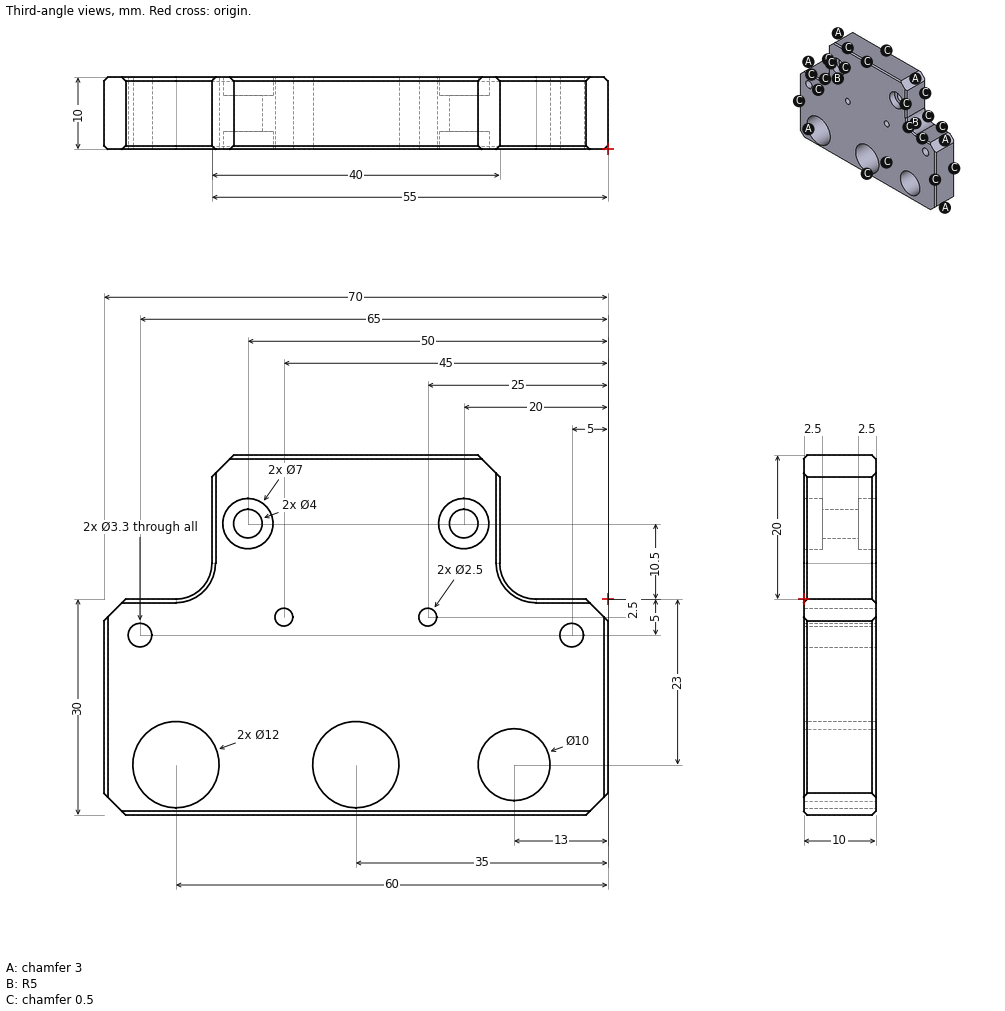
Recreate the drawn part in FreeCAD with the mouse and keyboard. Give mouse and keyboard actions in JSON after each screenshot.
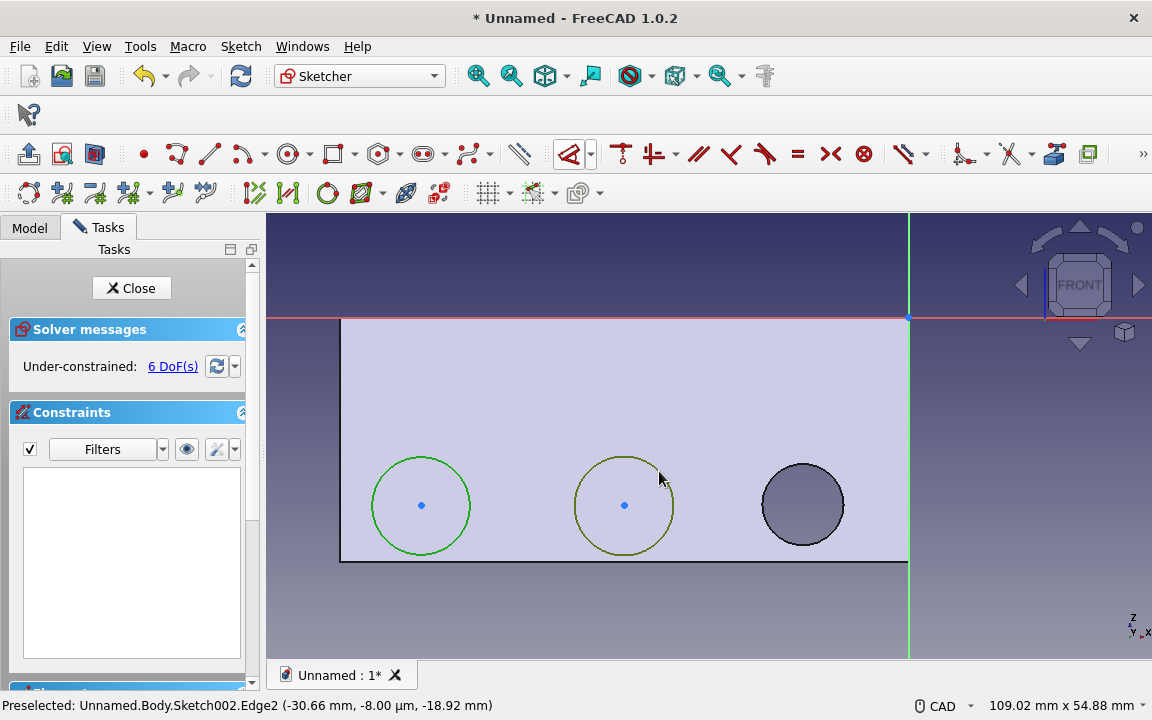
{"action": "left_click", "coordinate": [798, 154]}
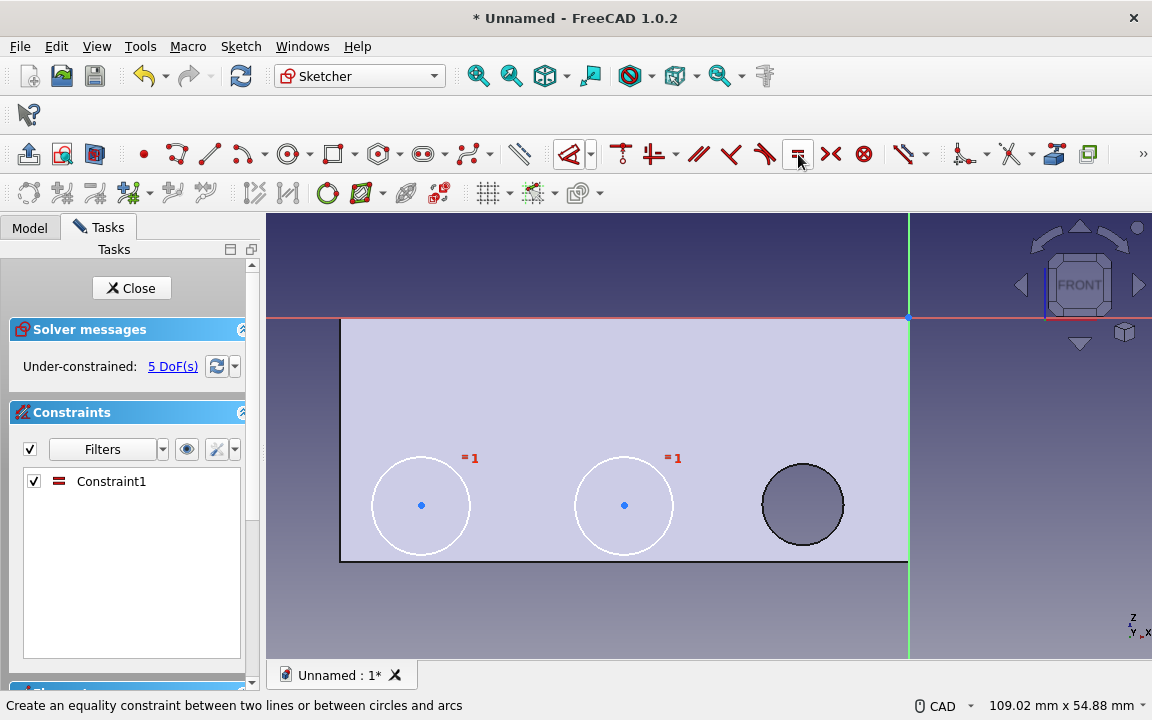
{"action": "left_click", "coordinate": [421, 506]}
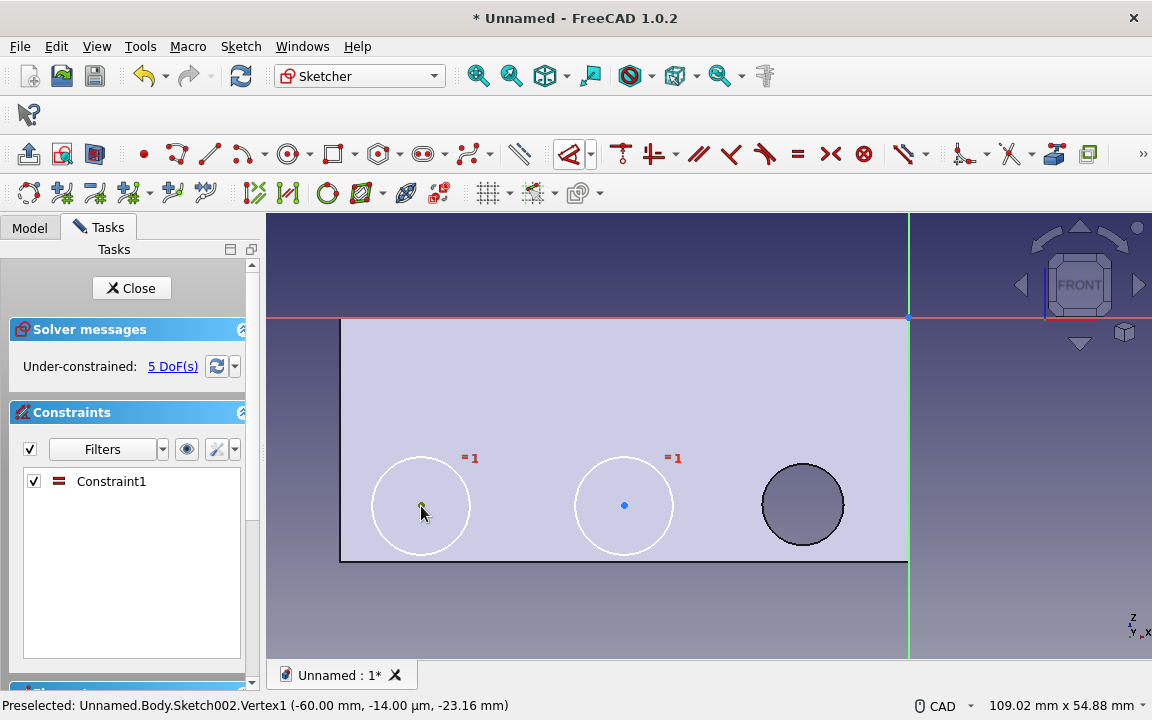
{"action": "left_click", "coordinate": [624, 506]}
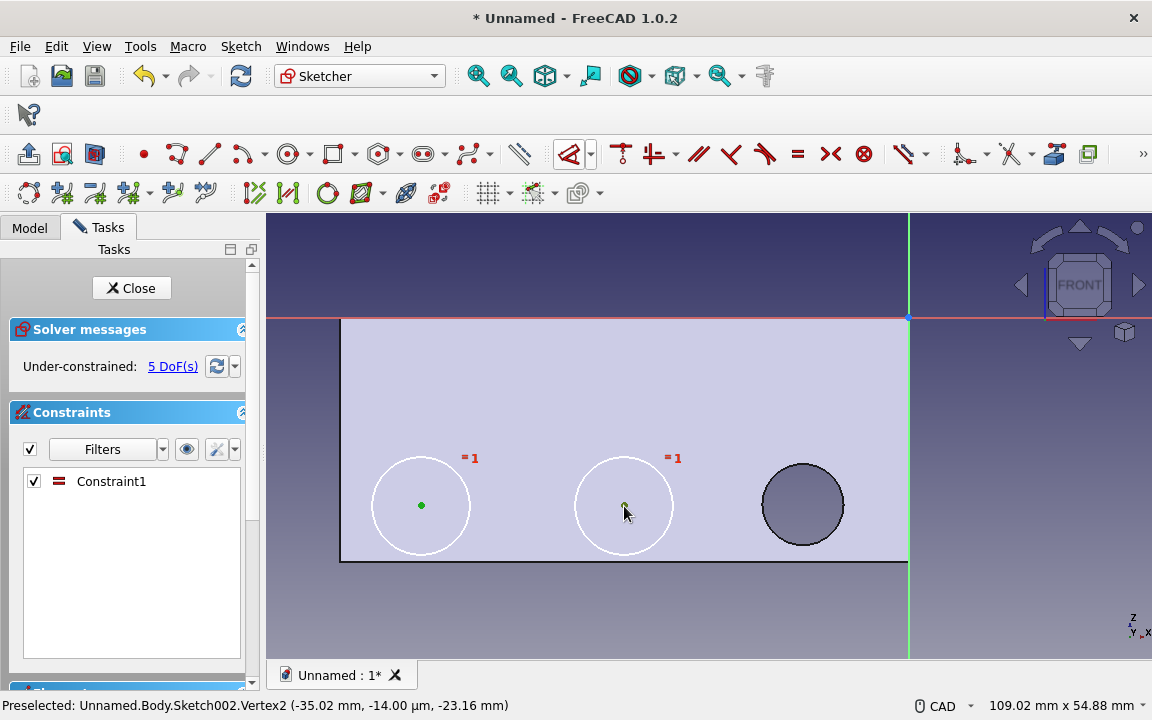
{"action": "left_click", "coordinate": [676, 154]}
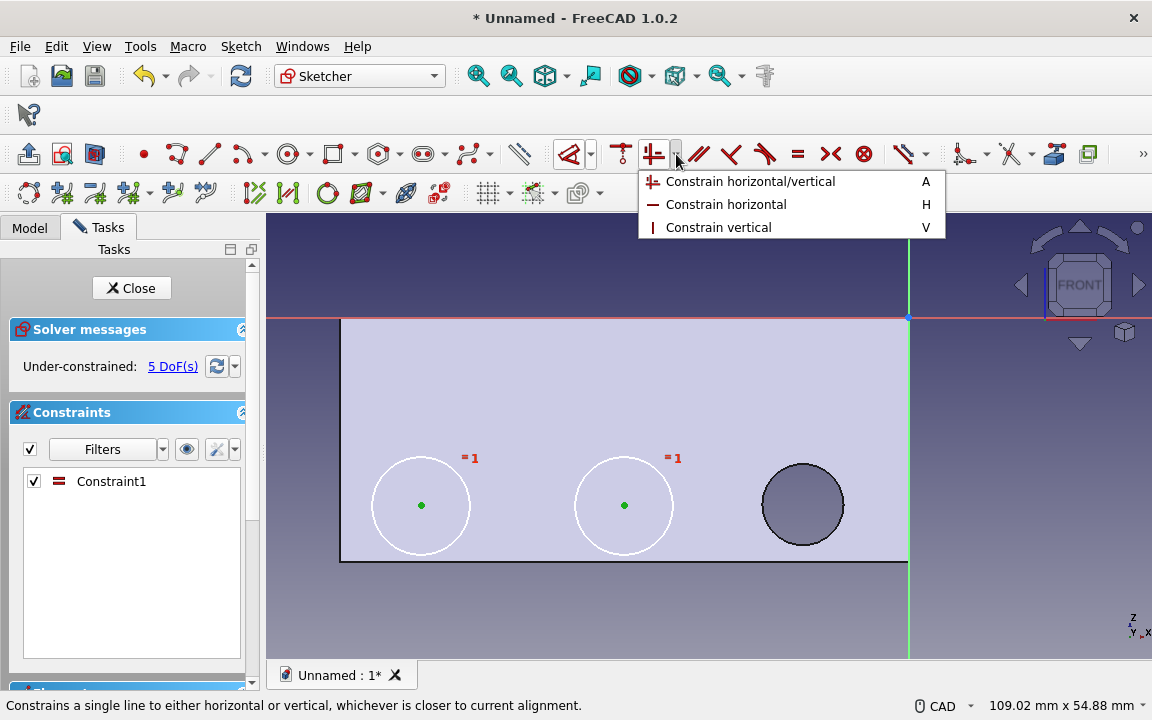
{"action": "left_click", "coordinate": [792, 204]}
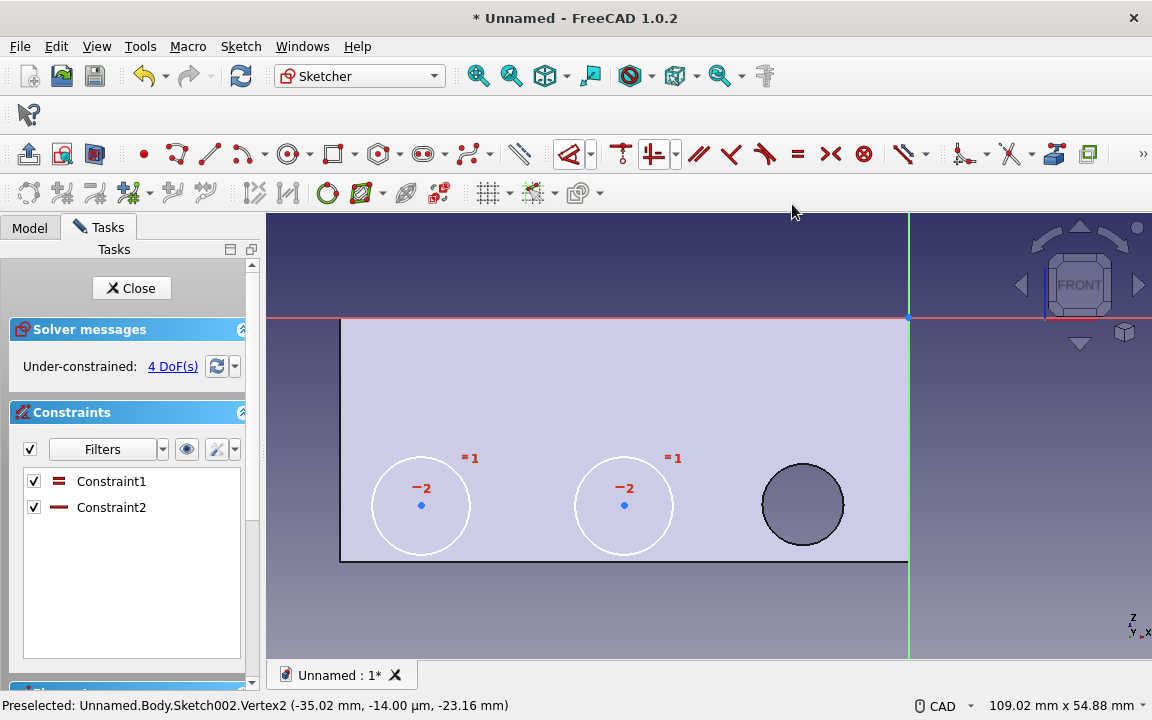
{"action": "left_click", "coordinate": [455, 471]}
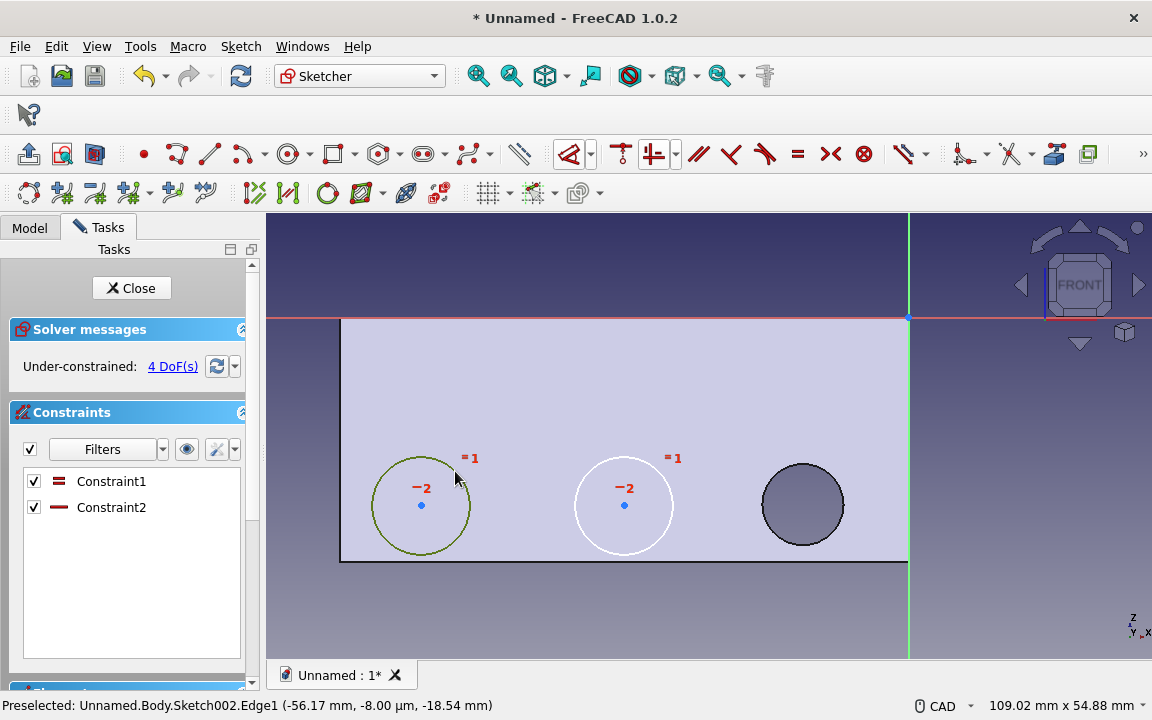
{"action": "left_click", "coordinate": [590, 154]}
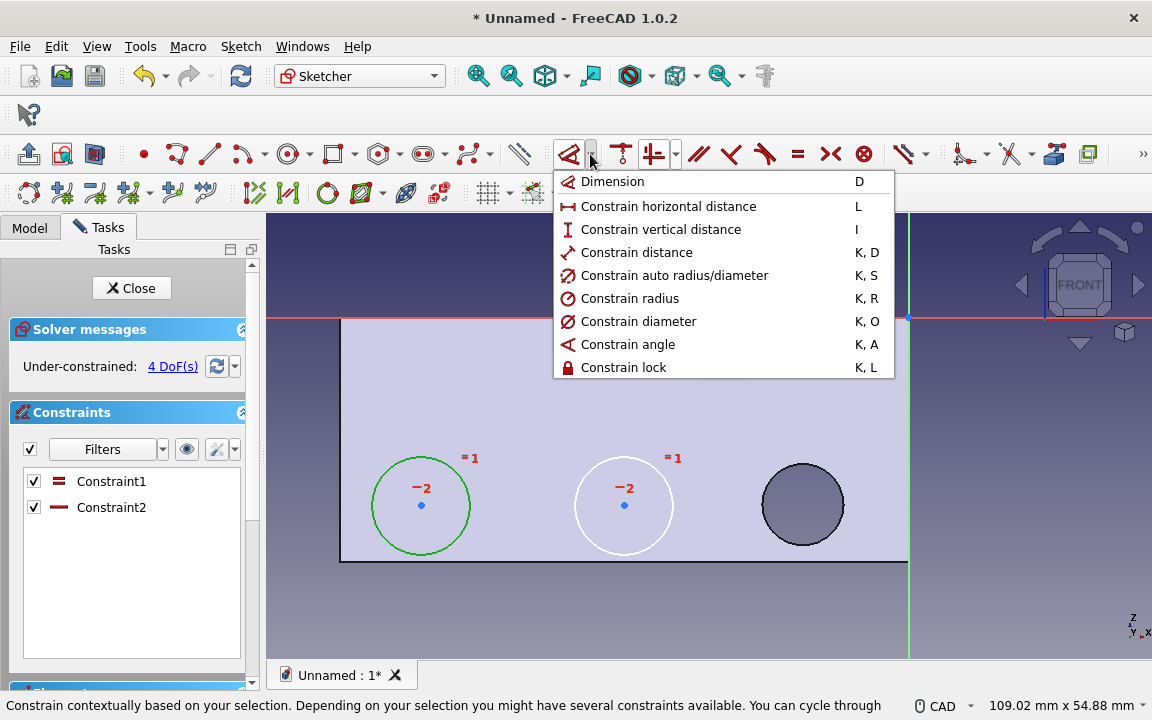
{"action": "left_click", "coordinate": [724, 322]}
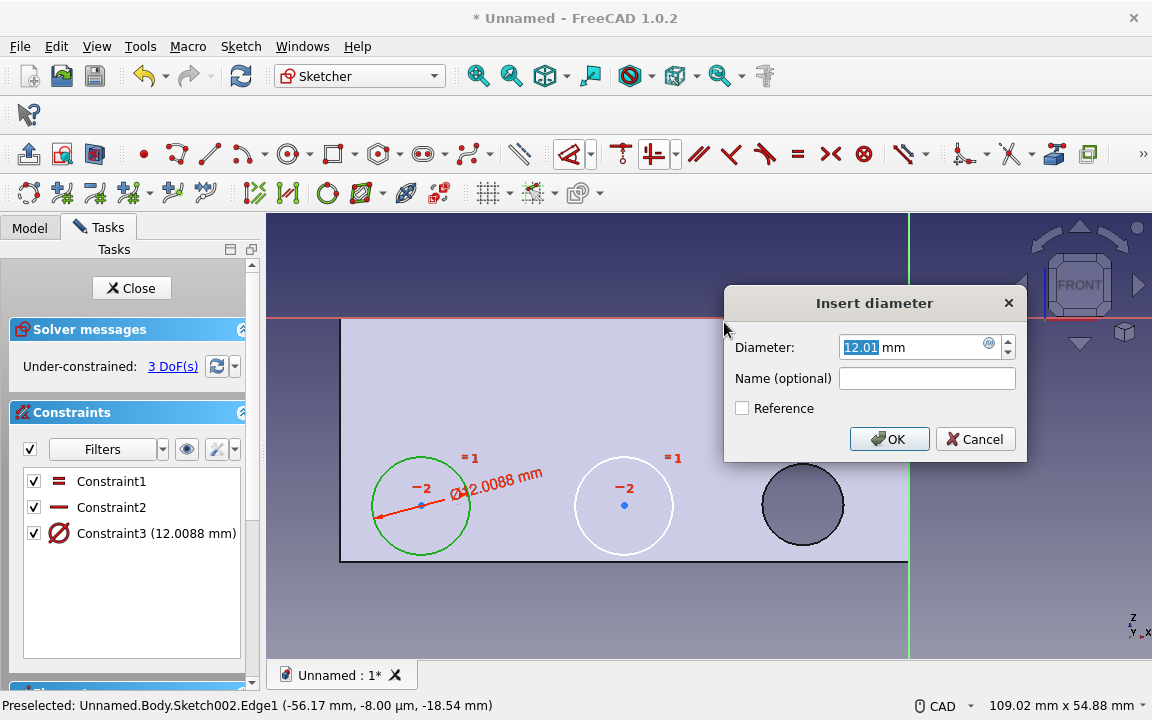
{"action": "type", "text": "12"}
{"action": "key", "text": "Return"}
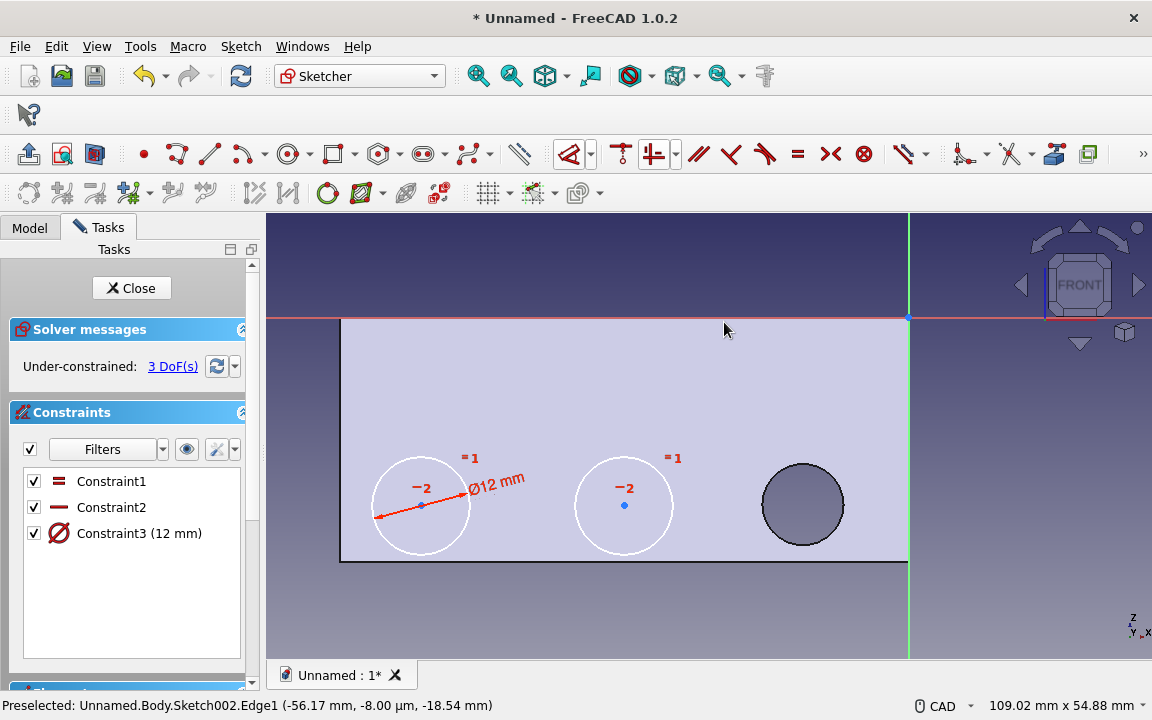
{"action": "left_click", "coordinate": [421, 506]}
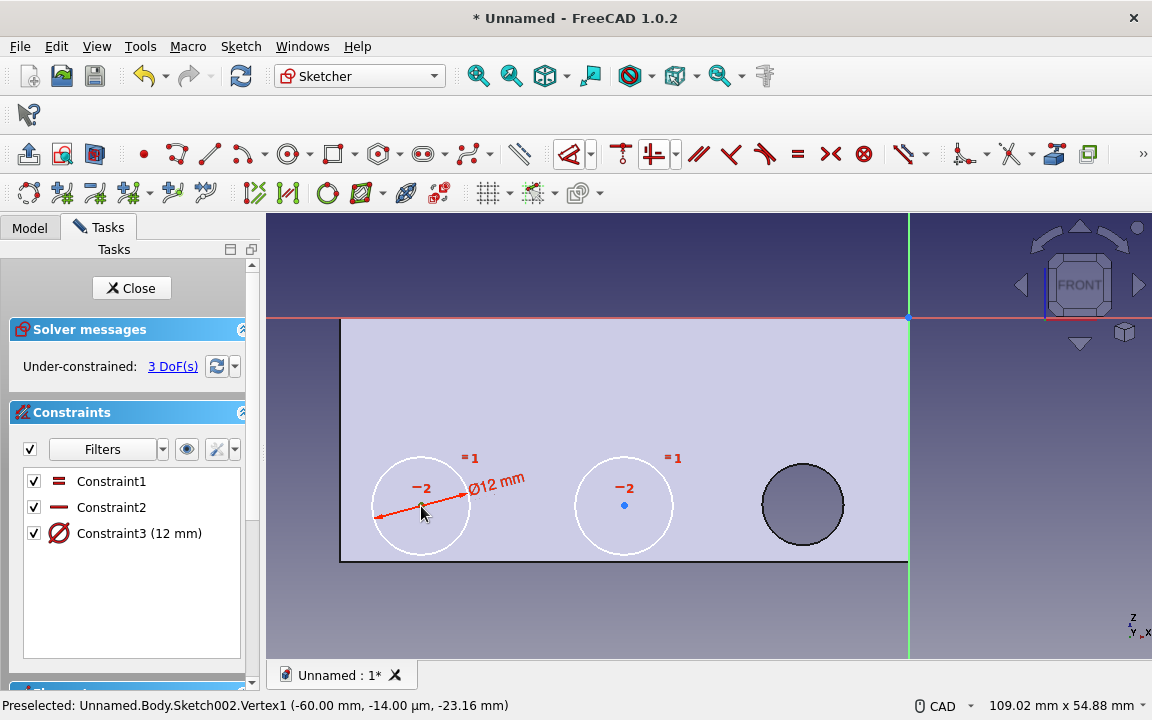
{"action": "left_click", "coordinate": [590, 154]}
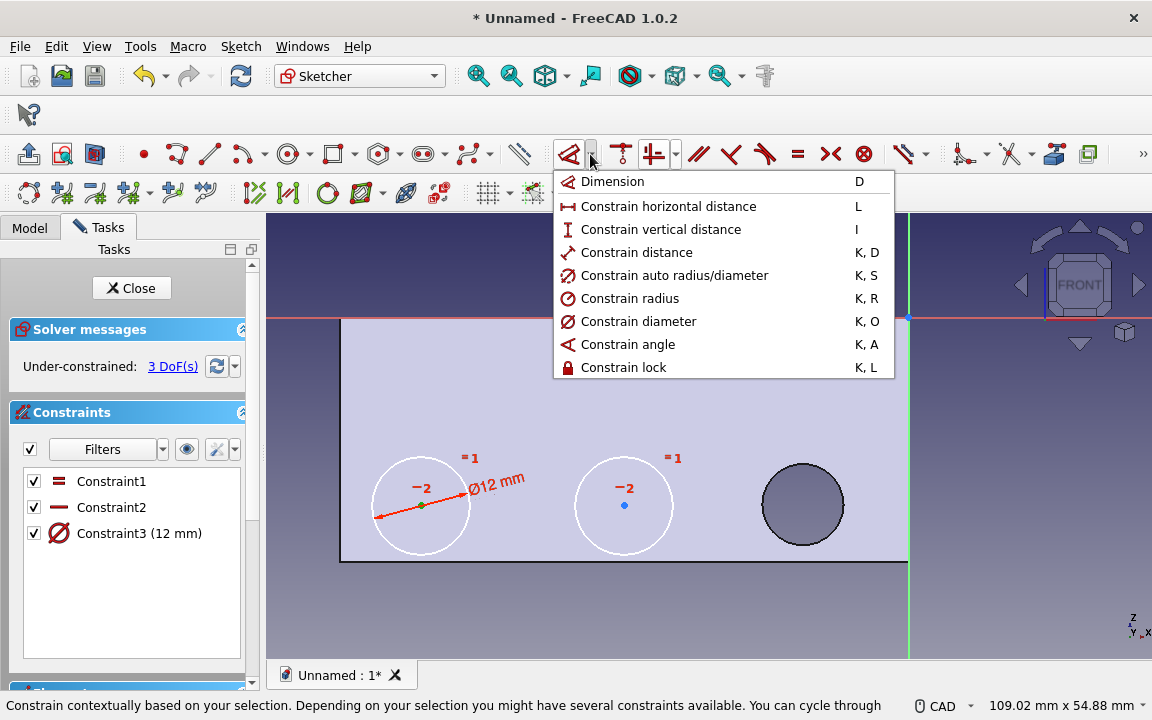
{"action": "left_click", "coordinate": [724, 206]}